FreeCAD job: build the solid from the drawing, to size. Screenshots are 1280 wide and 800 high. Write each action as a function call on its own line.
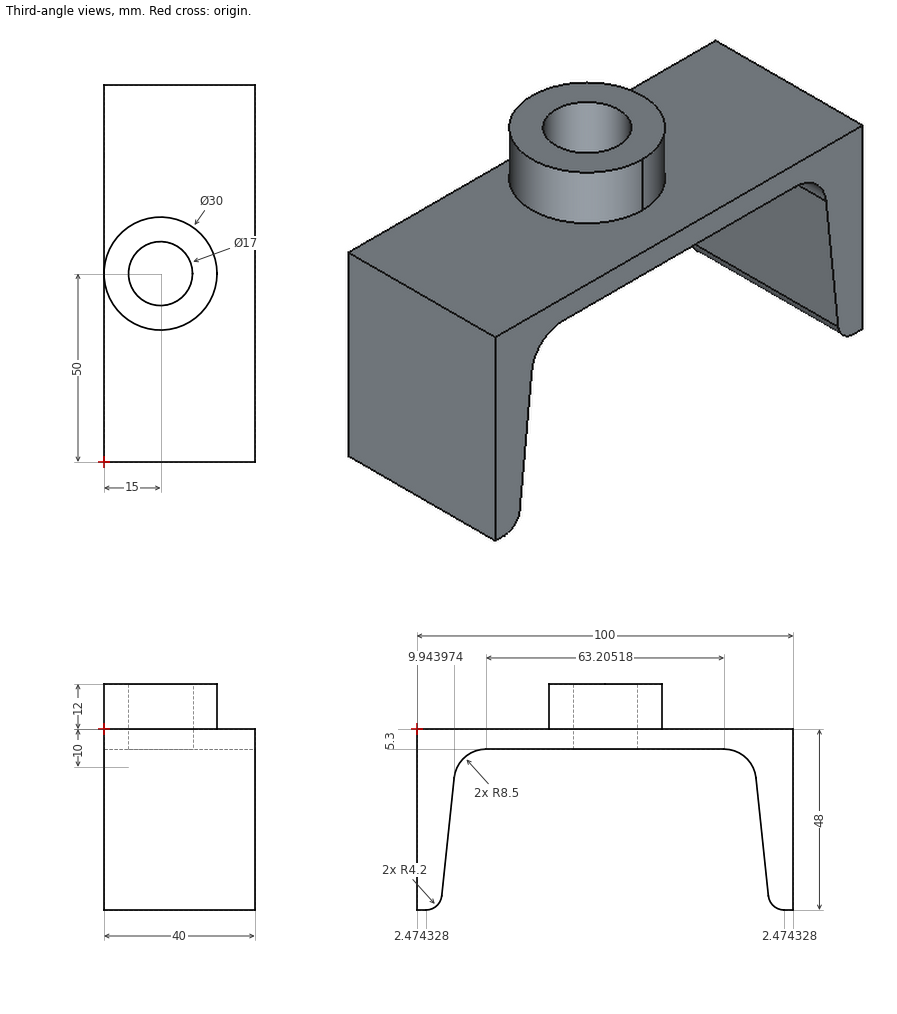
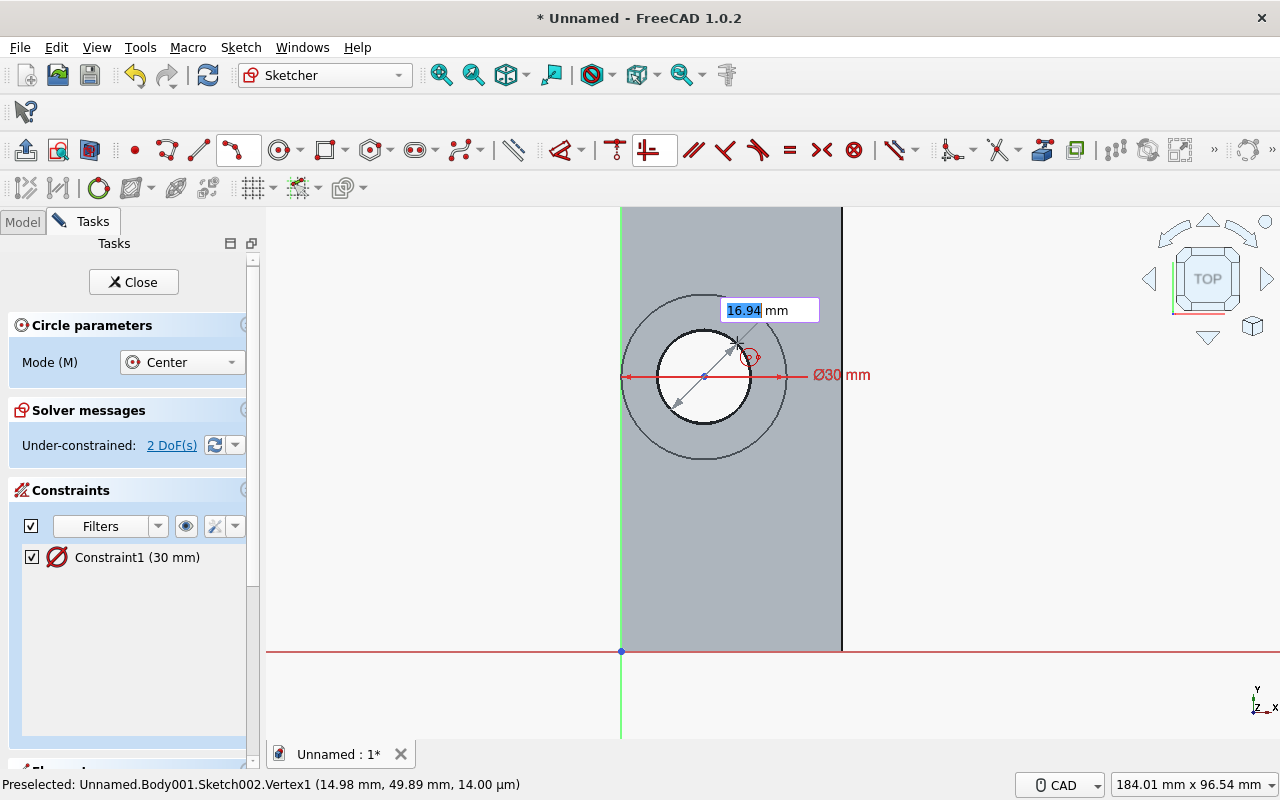
text(17)
key(Return)
key(Escape)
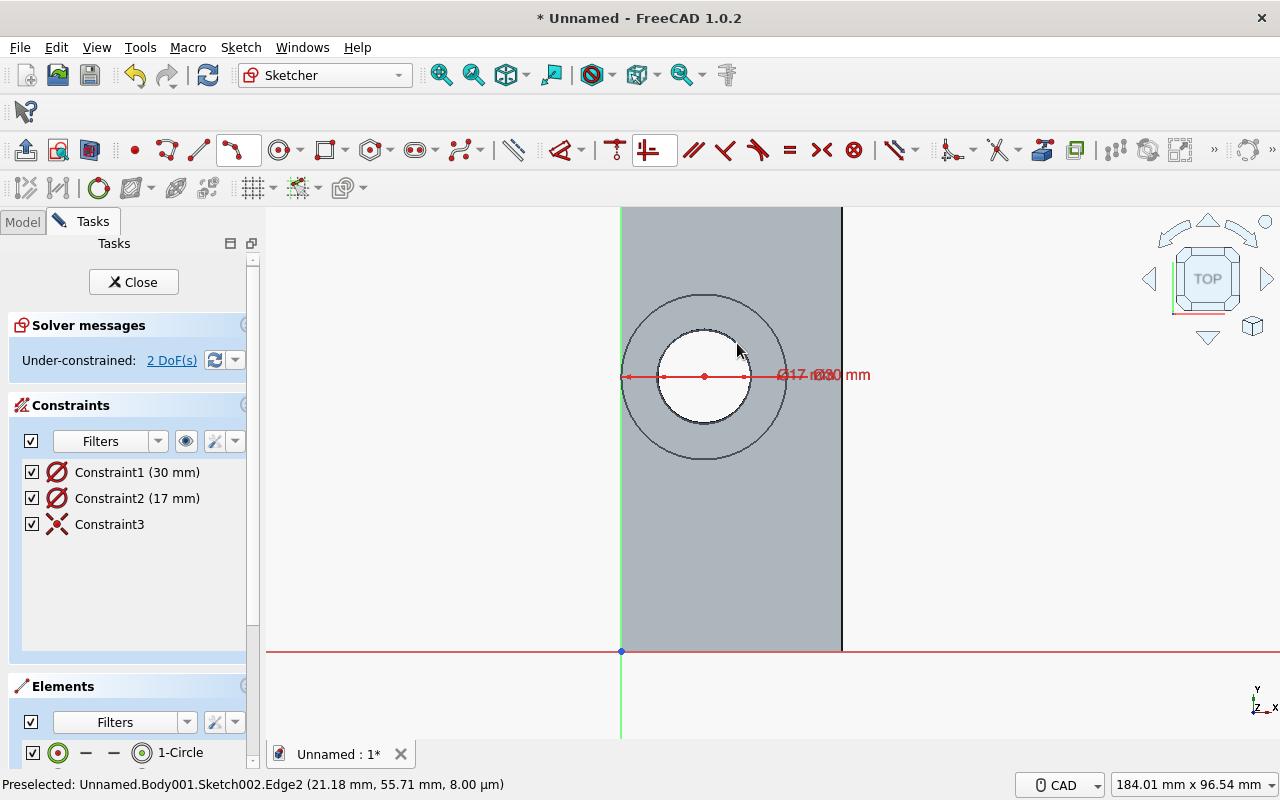
click(560, 150)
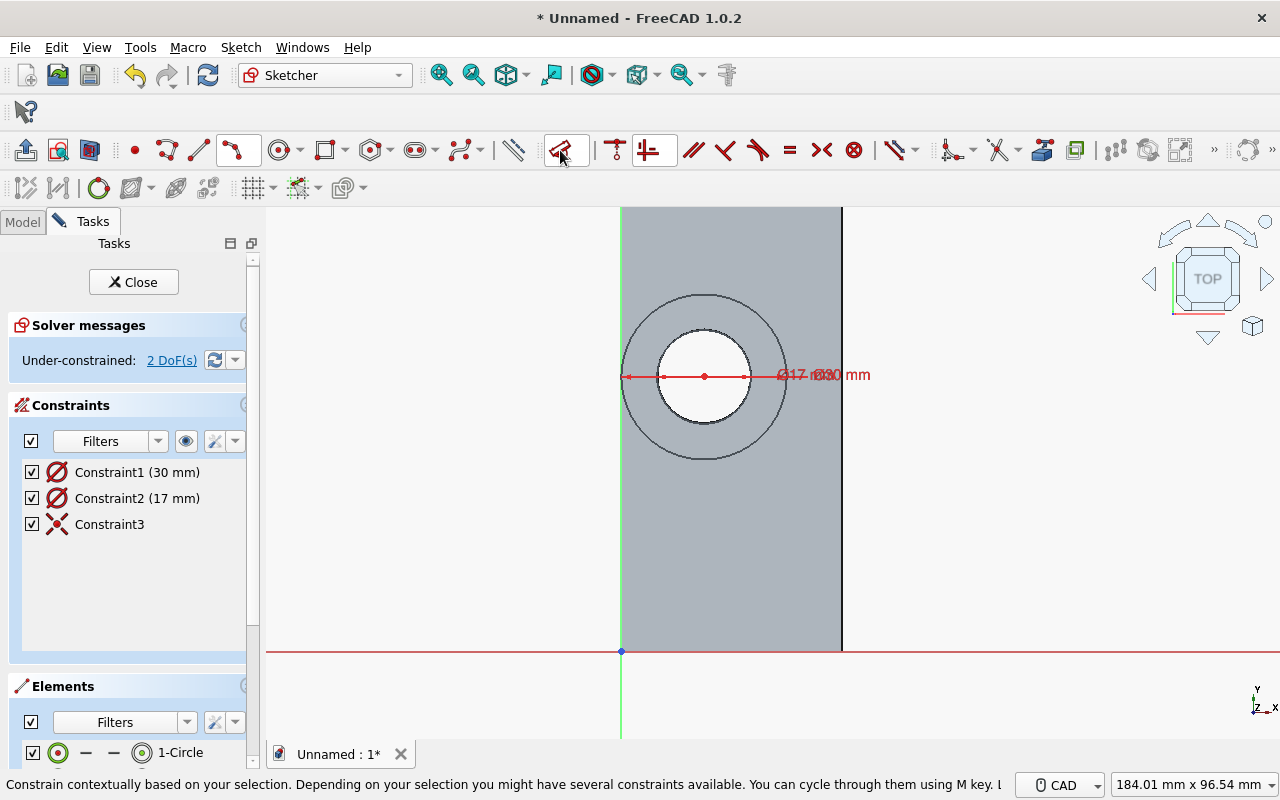
click(704, 377)
click(663, 686)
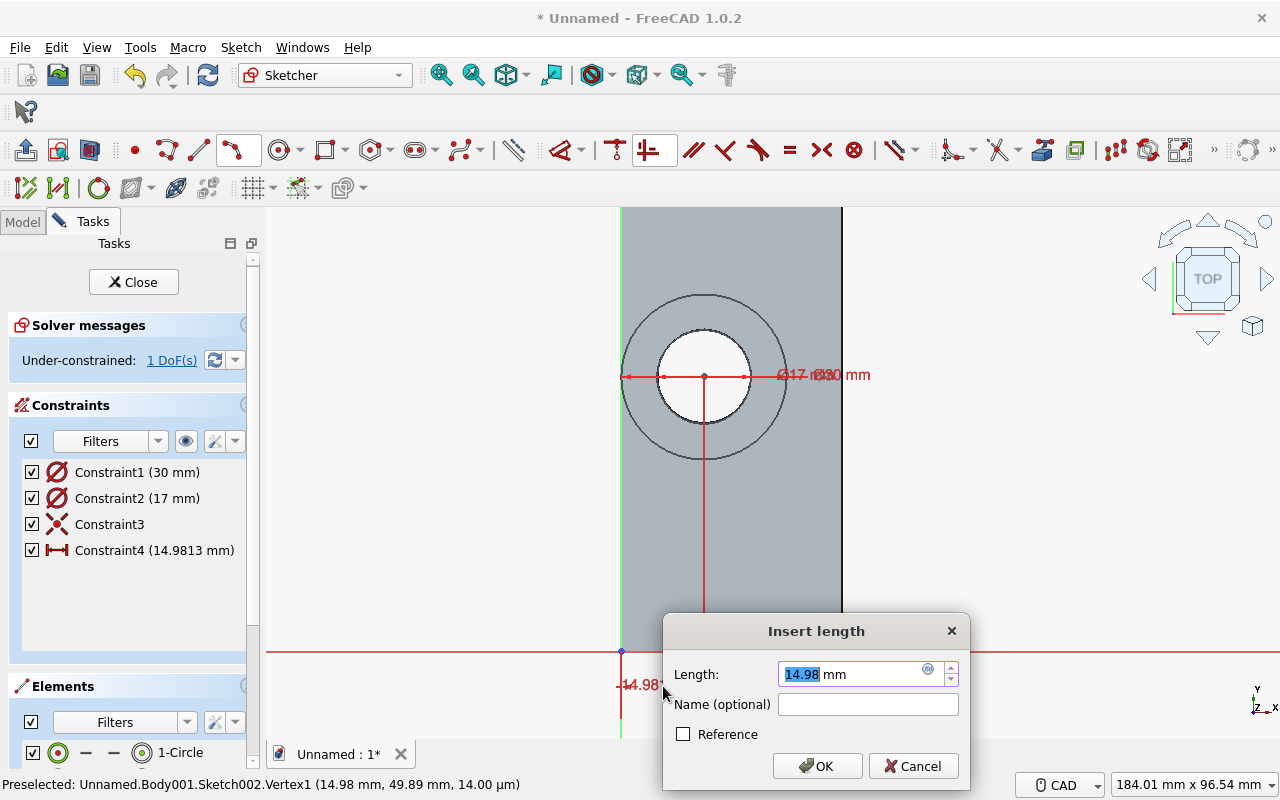
text(15)
key(Return)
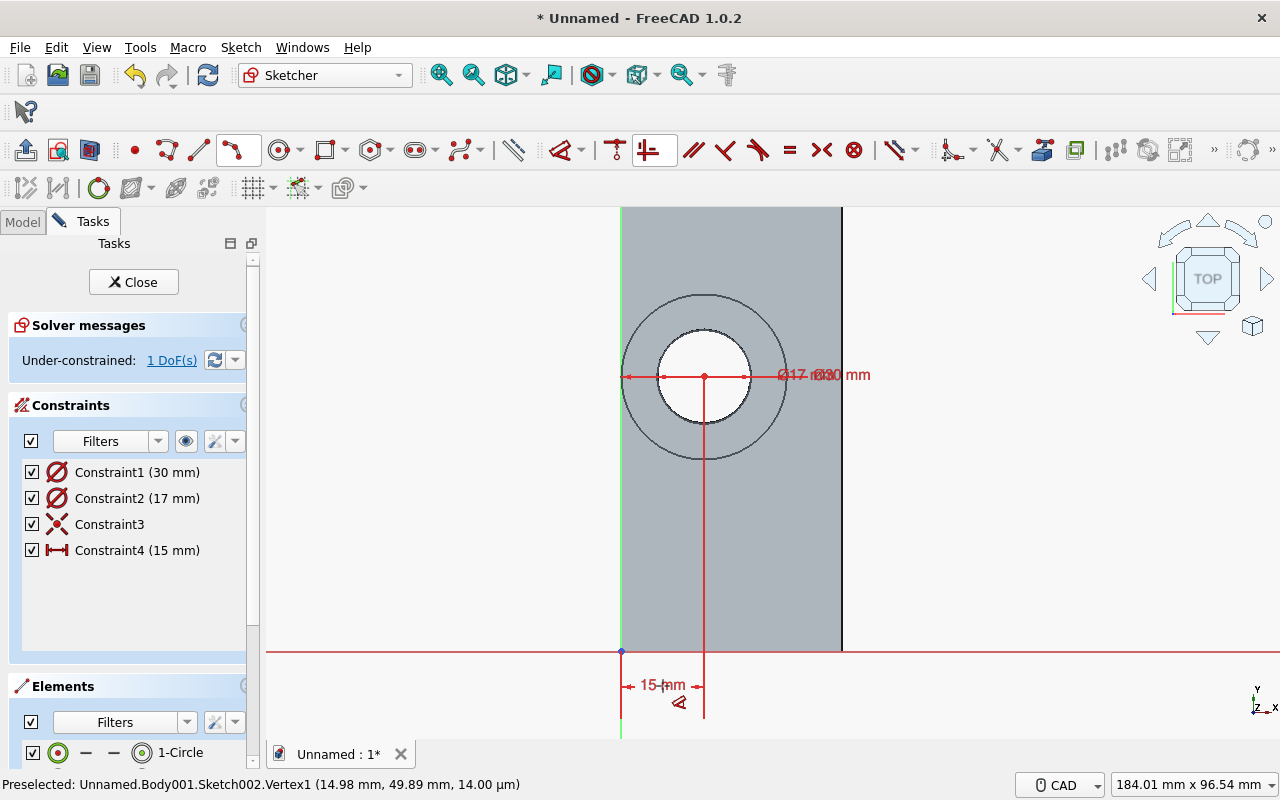
click(704, 377)
click(587, 514)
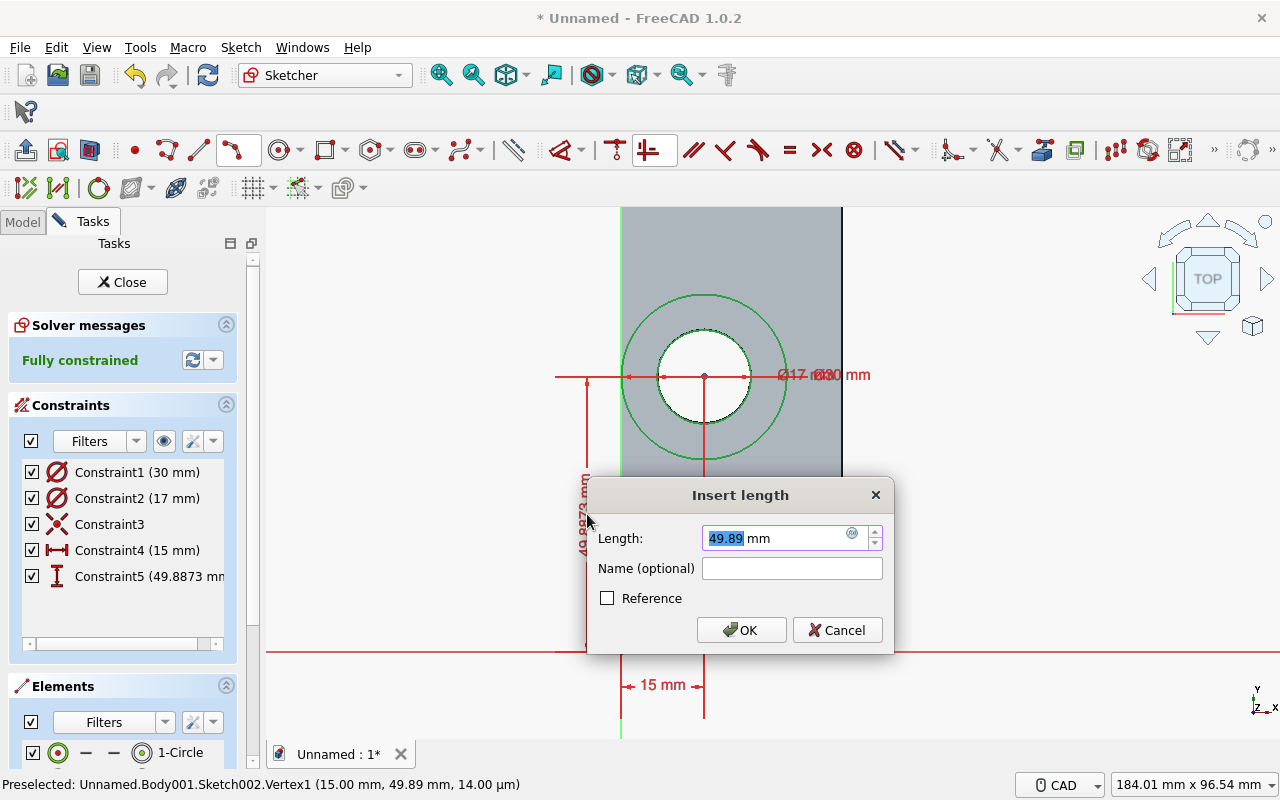
text(50)
key(Return)
key(Escape)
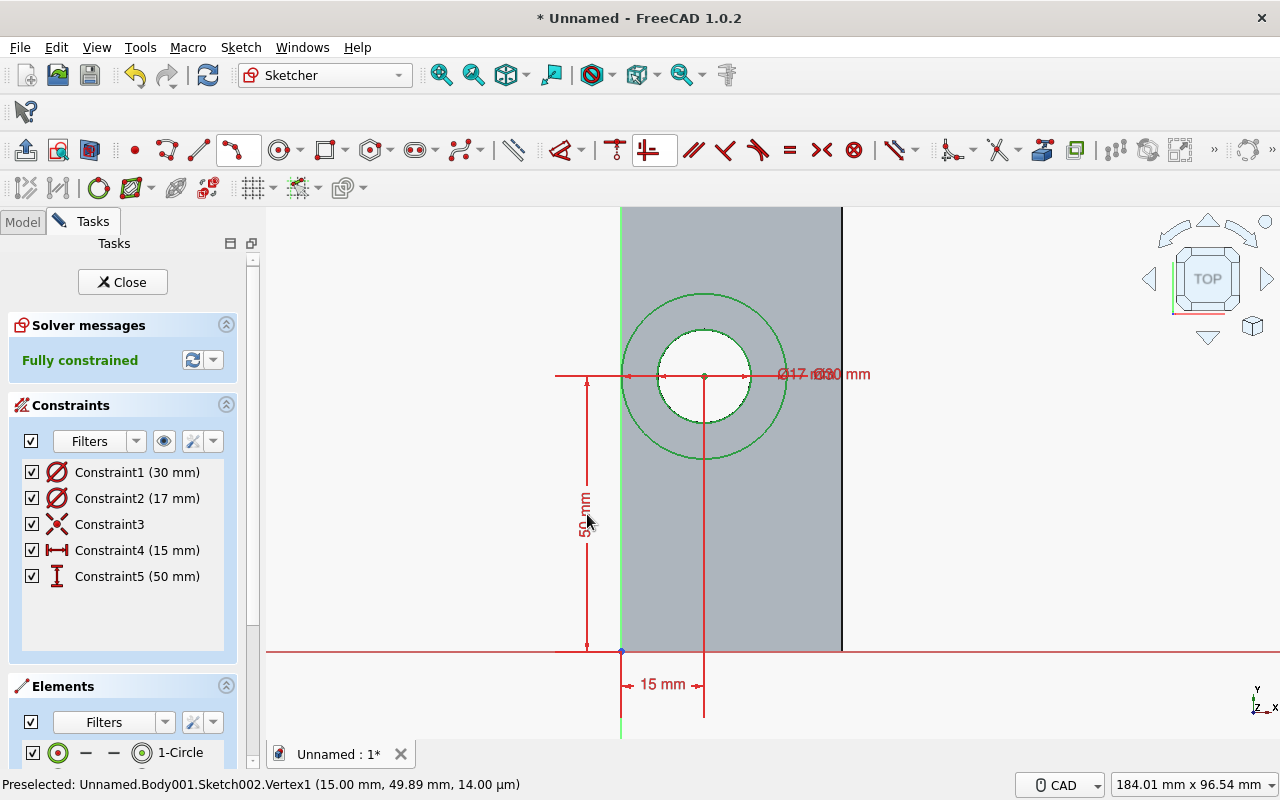
click(123, 282)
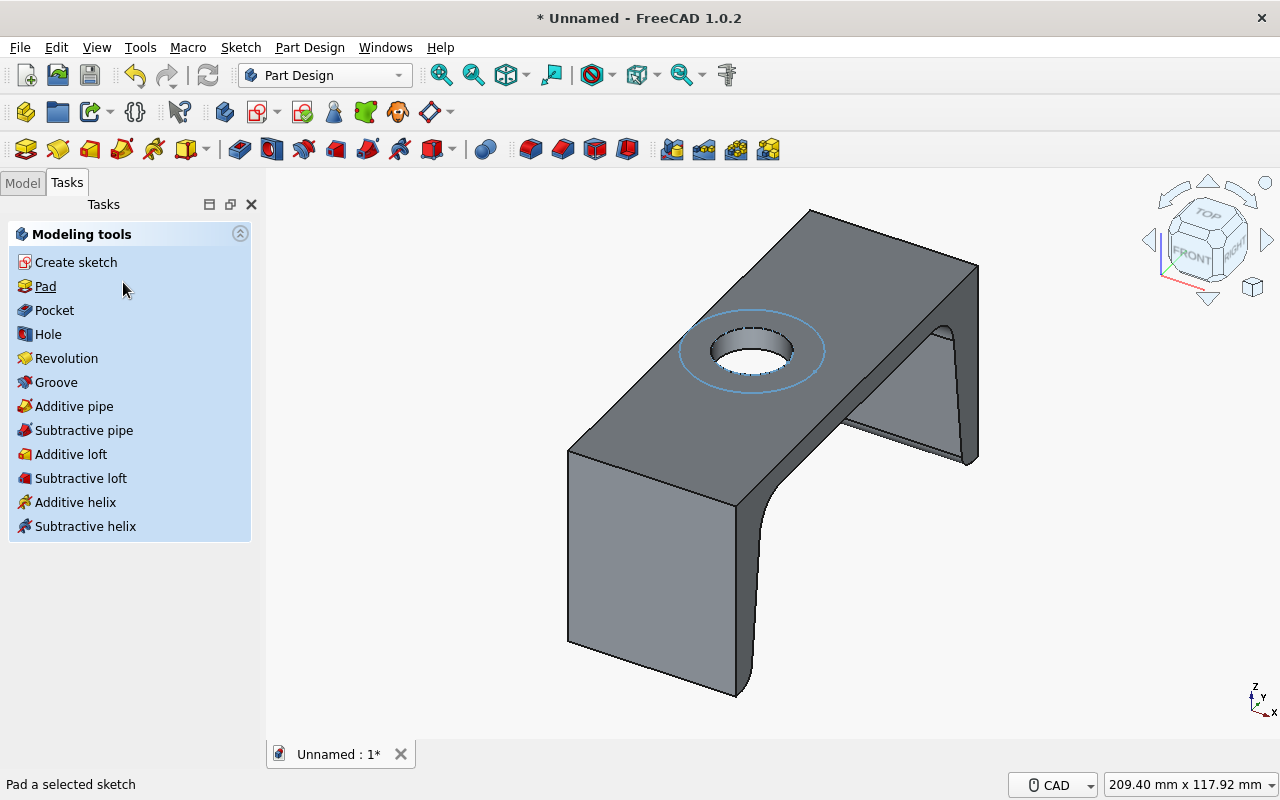
click(26, 150)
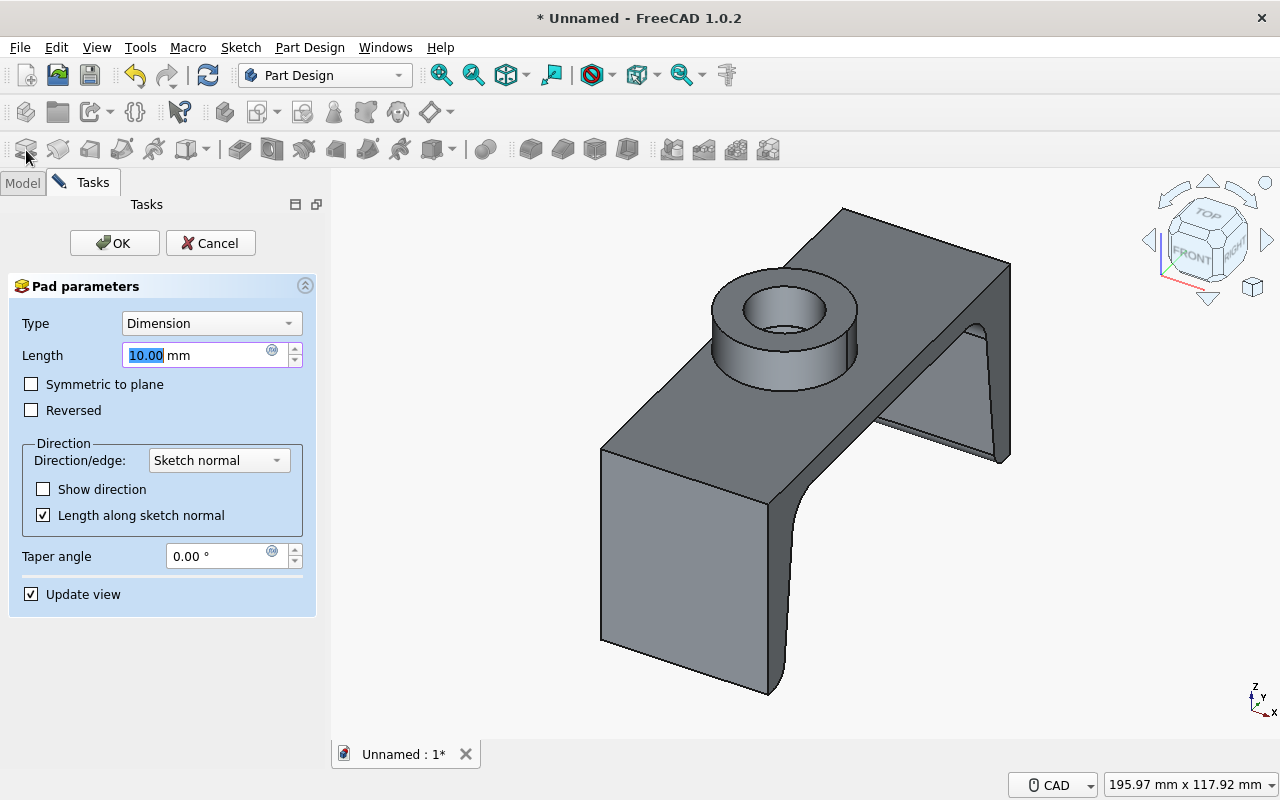
text(12)
key(Tab)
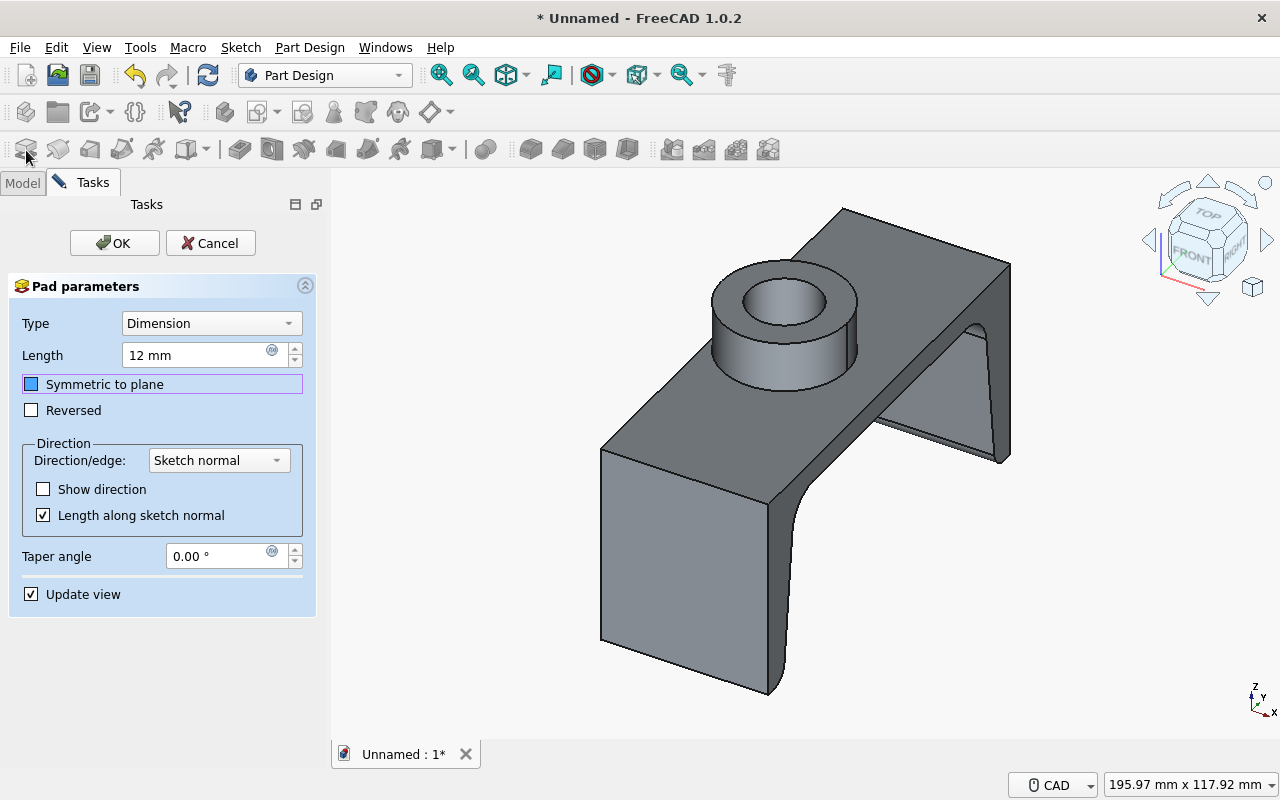
click(115, 243)